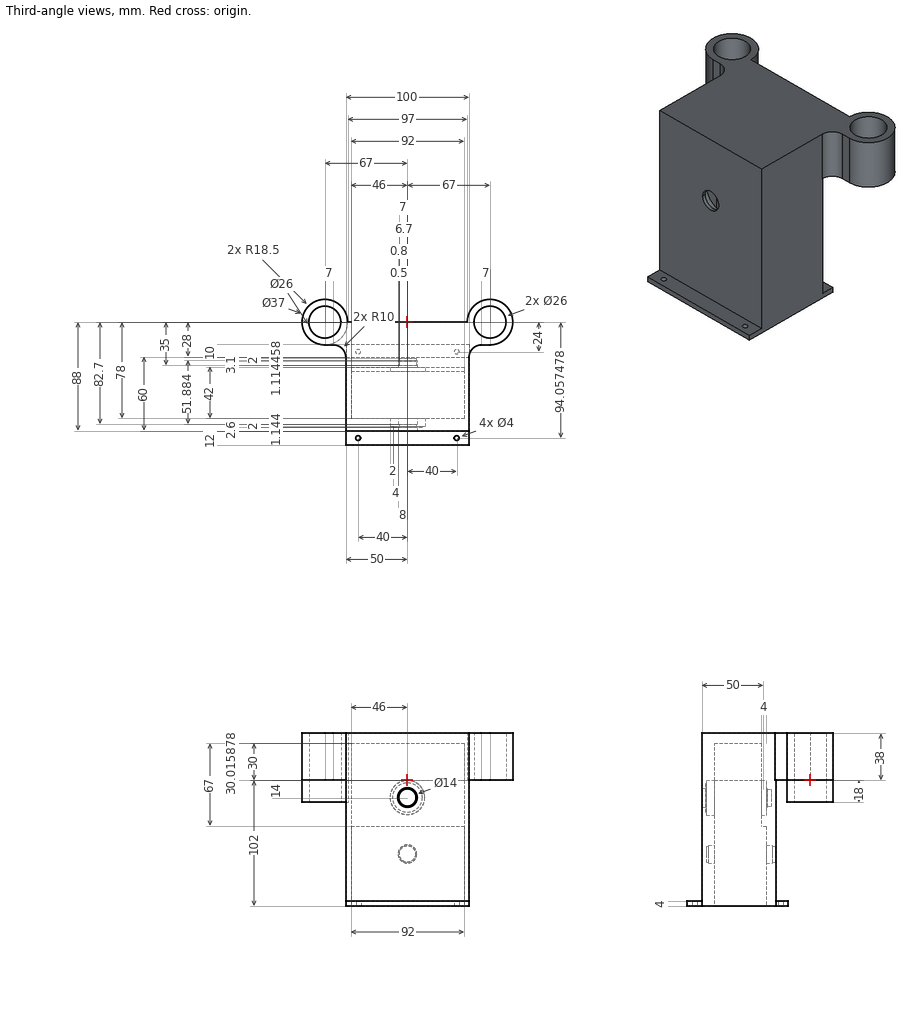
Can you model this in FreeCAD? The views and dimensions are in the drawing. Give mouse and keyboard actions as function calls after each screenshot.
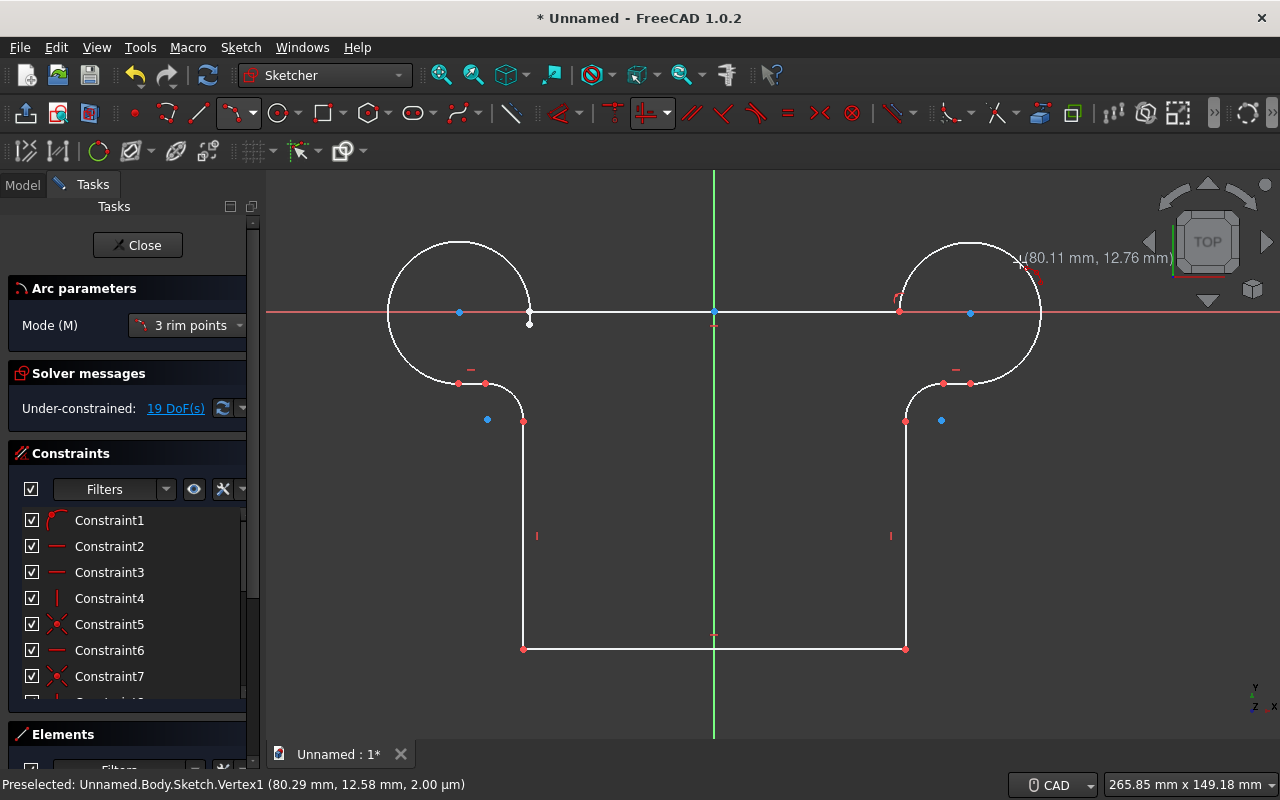
click(278, 114)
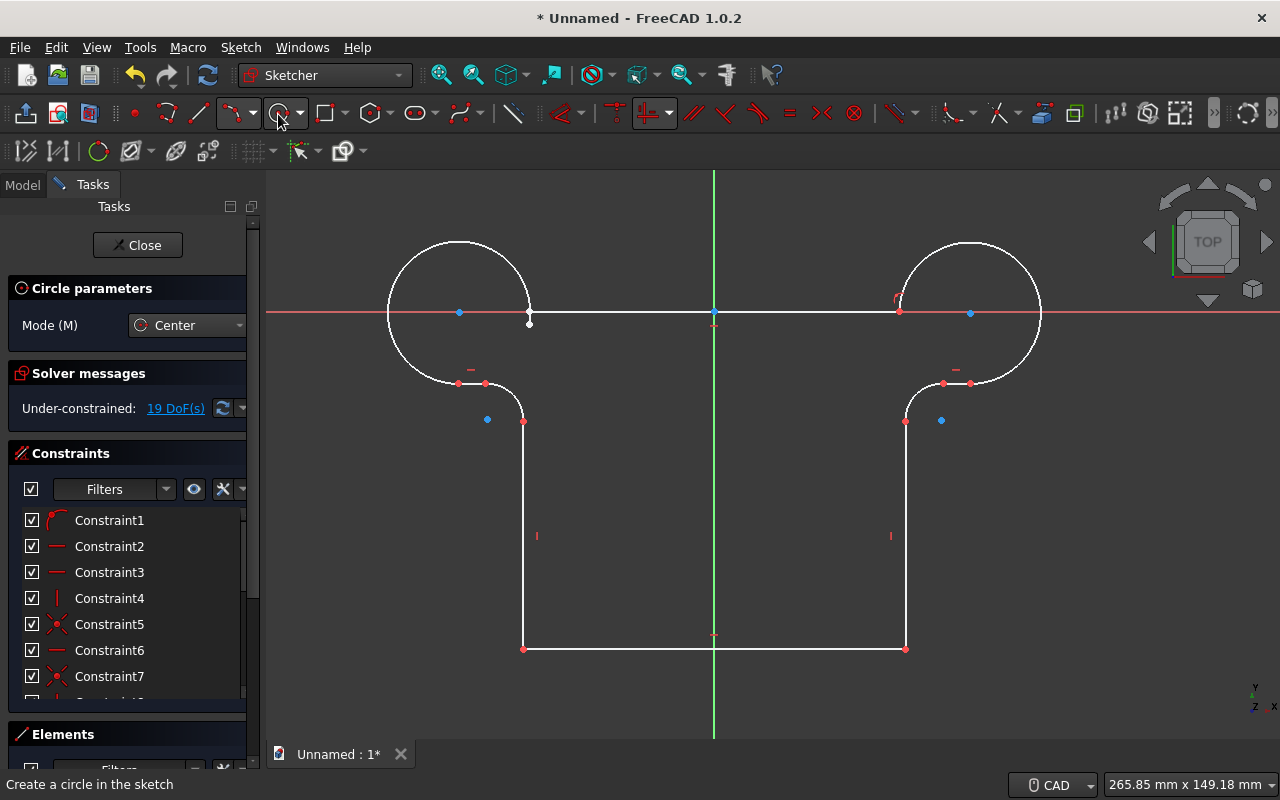
click(970, 312)
click(1005, 277)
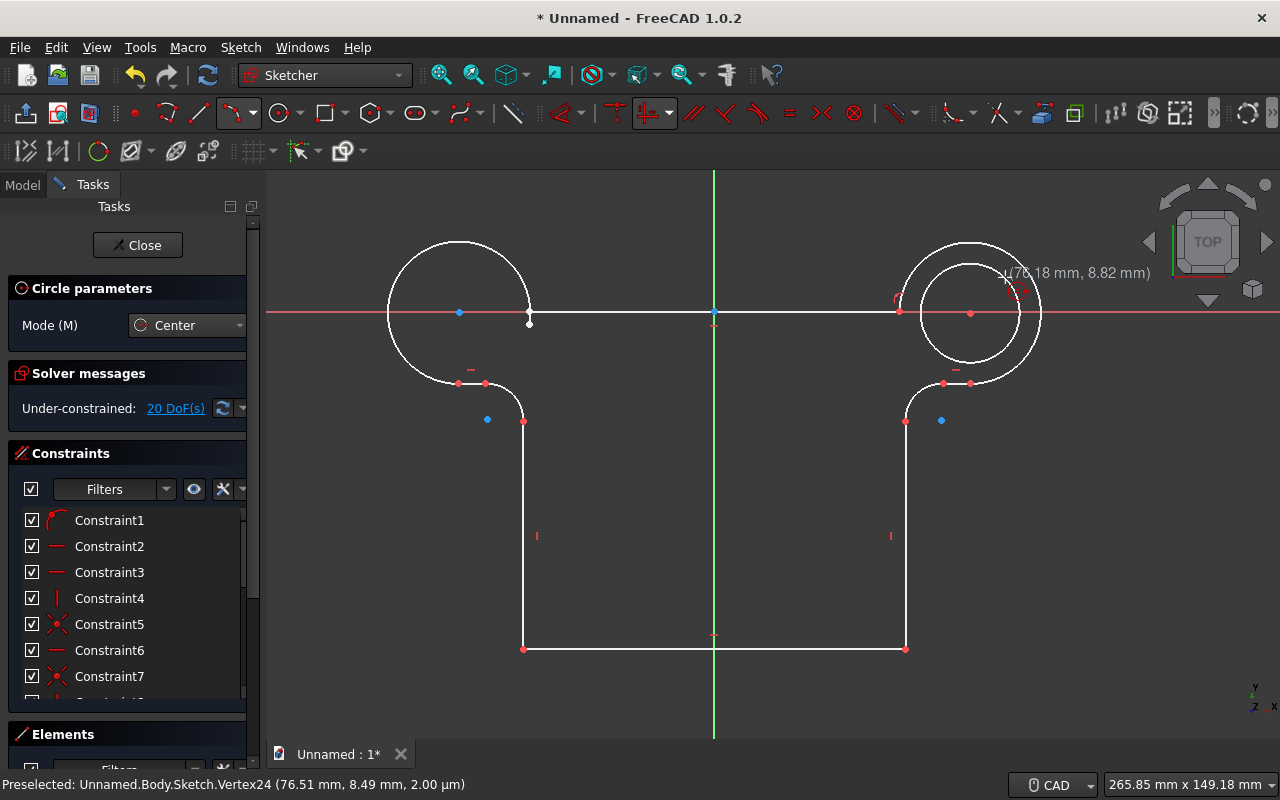
click(459, 312)
click(494, 277)
key(Escape)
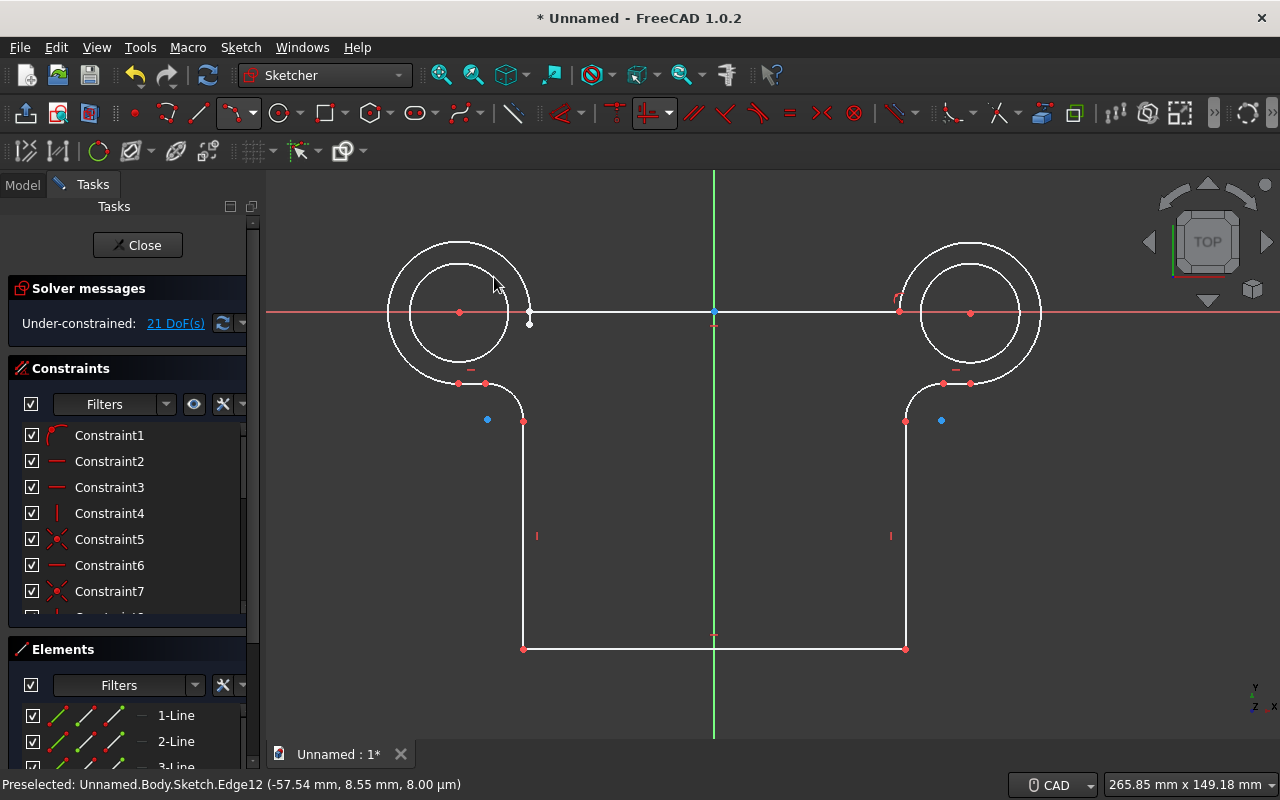
scroll(469, 384, up, 2)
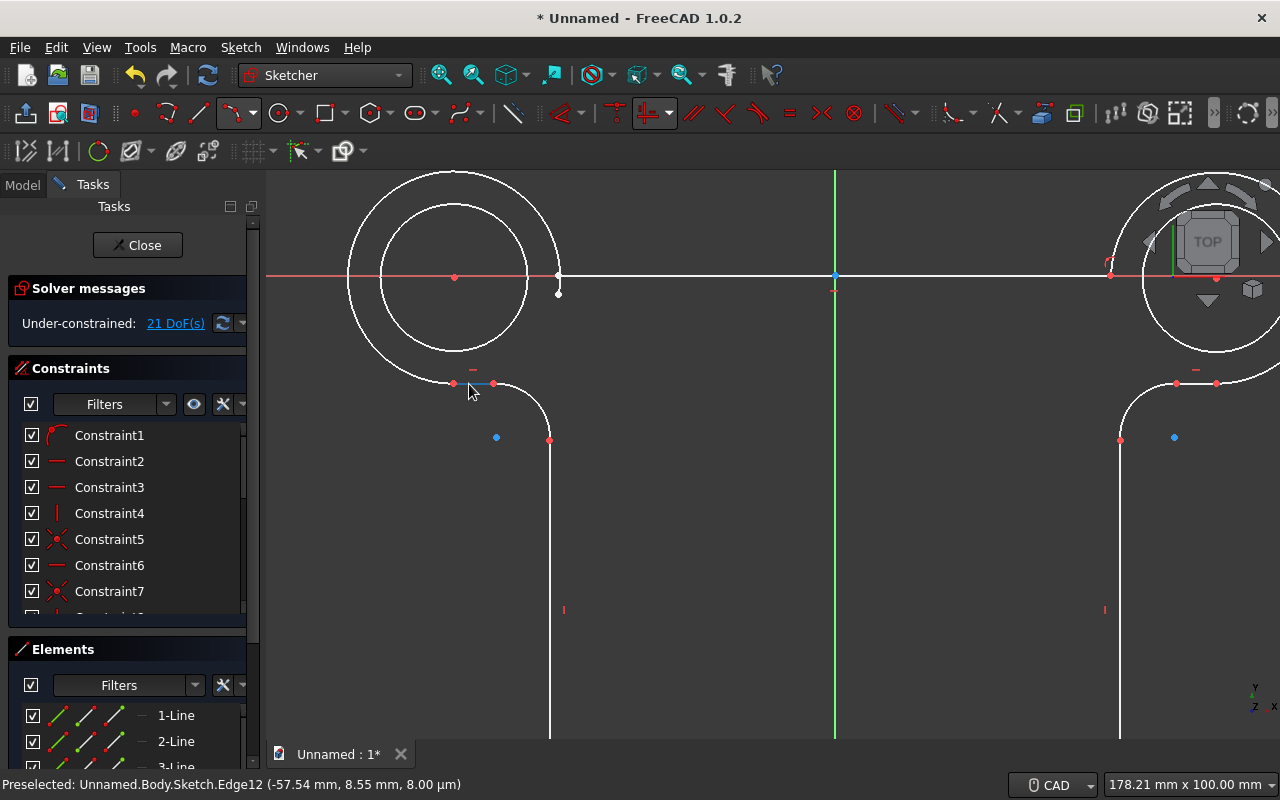
click(469, 384)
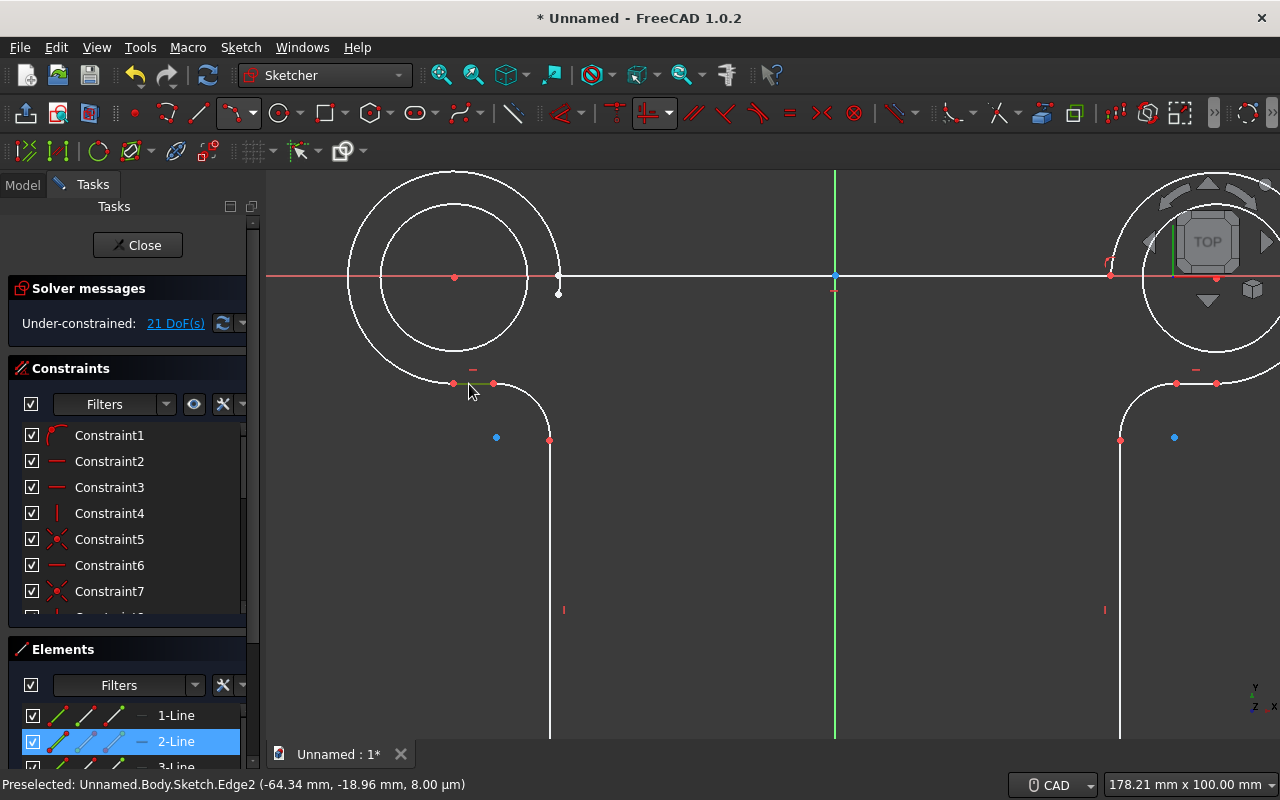
click(348, 289)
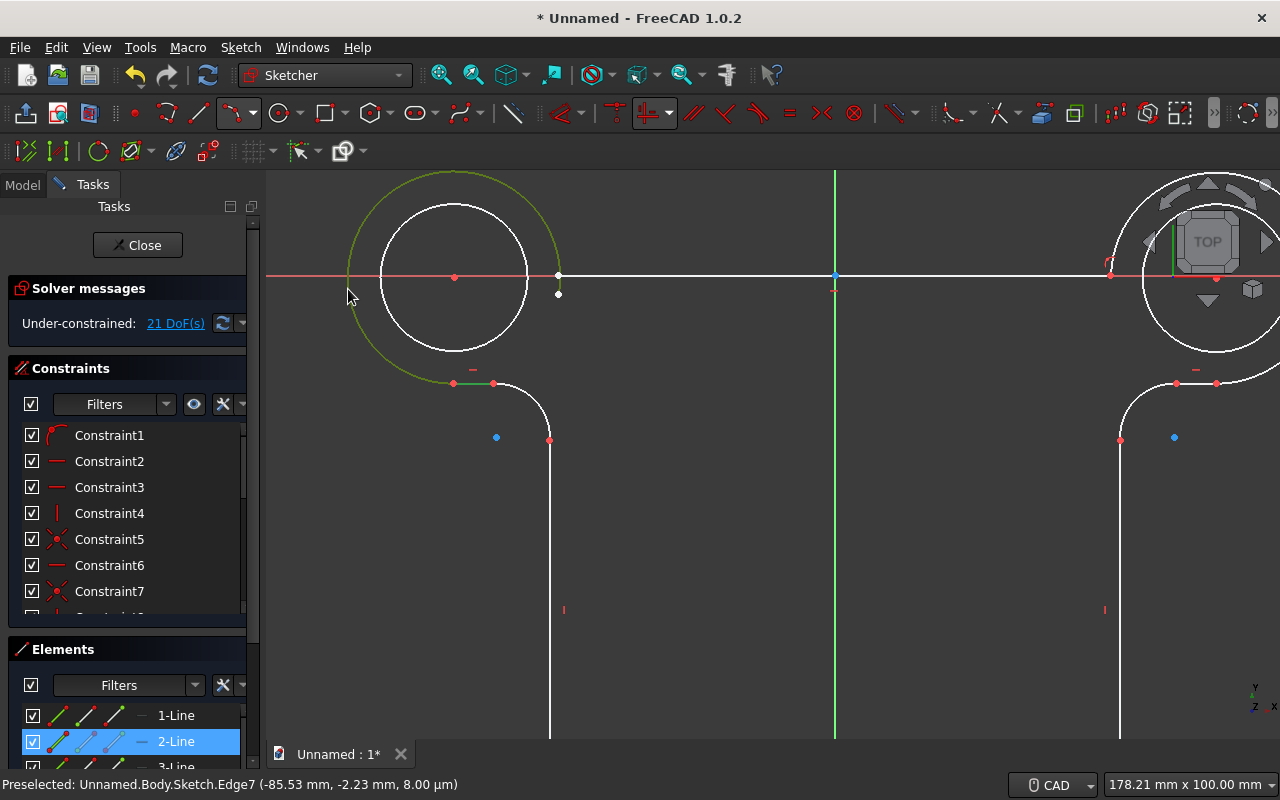
key(t)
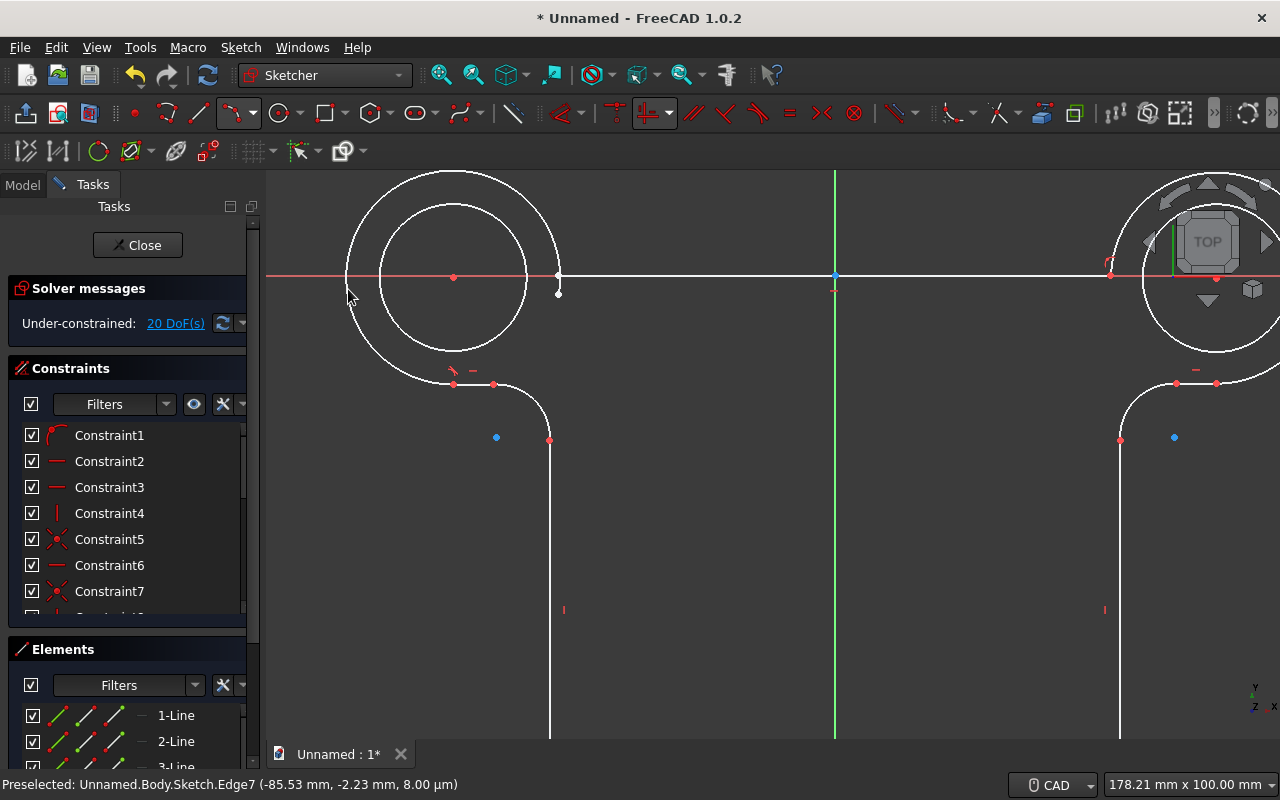
click(465, 385)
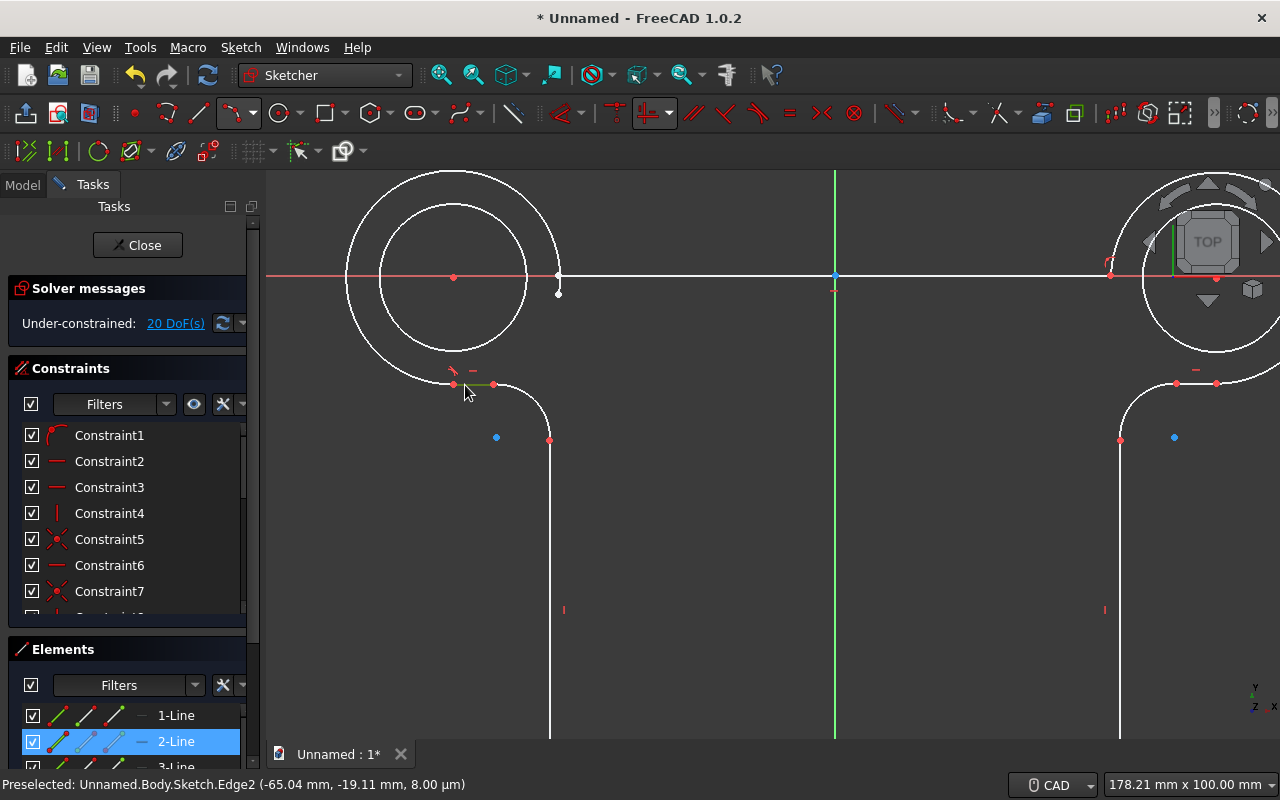
click(544, 414)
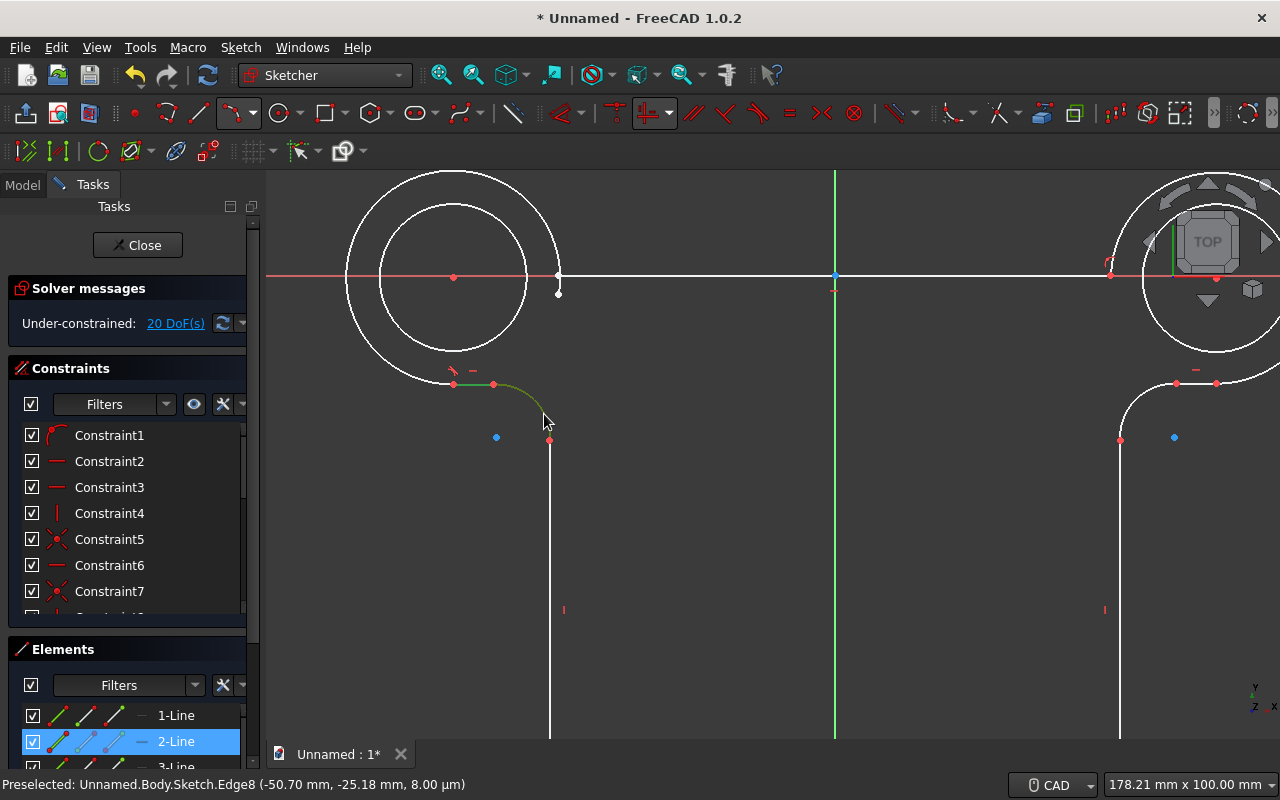
click(758, 114)